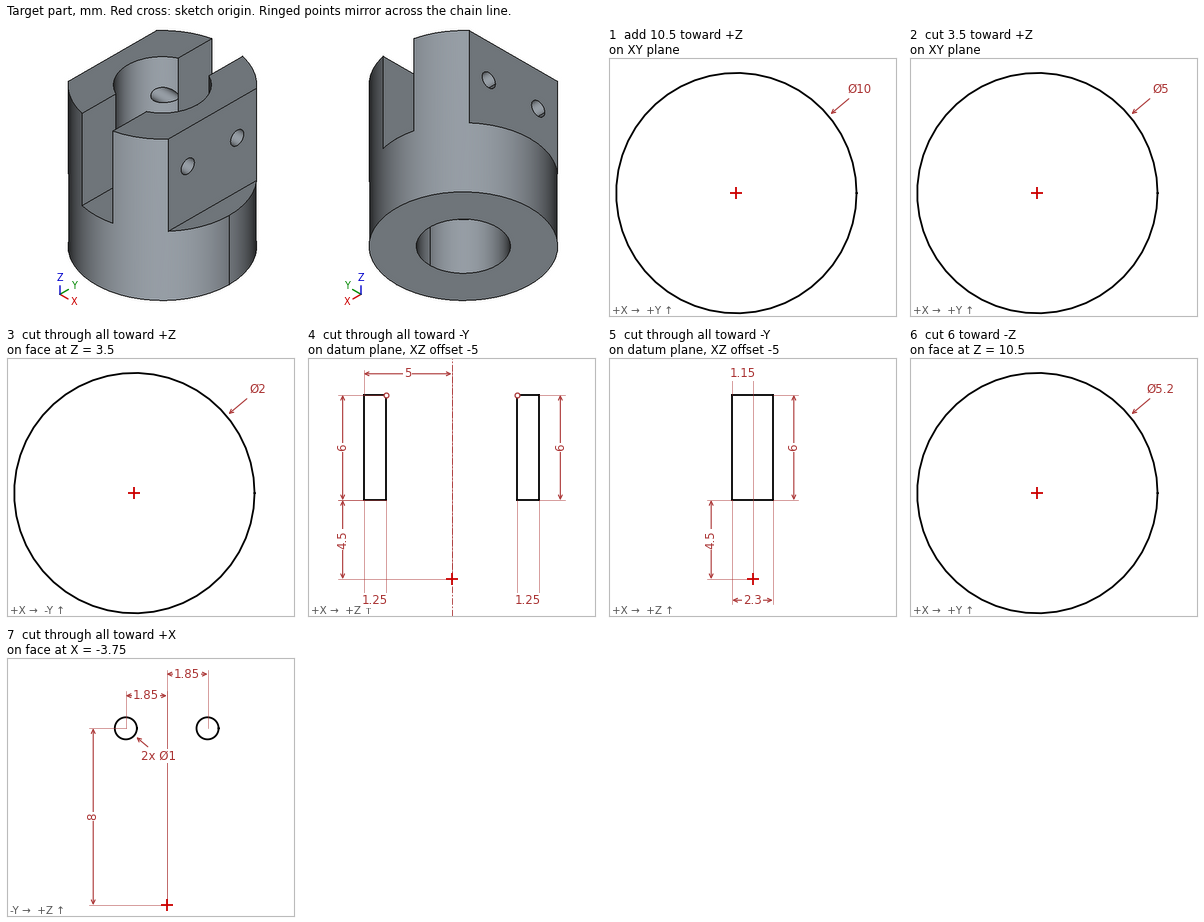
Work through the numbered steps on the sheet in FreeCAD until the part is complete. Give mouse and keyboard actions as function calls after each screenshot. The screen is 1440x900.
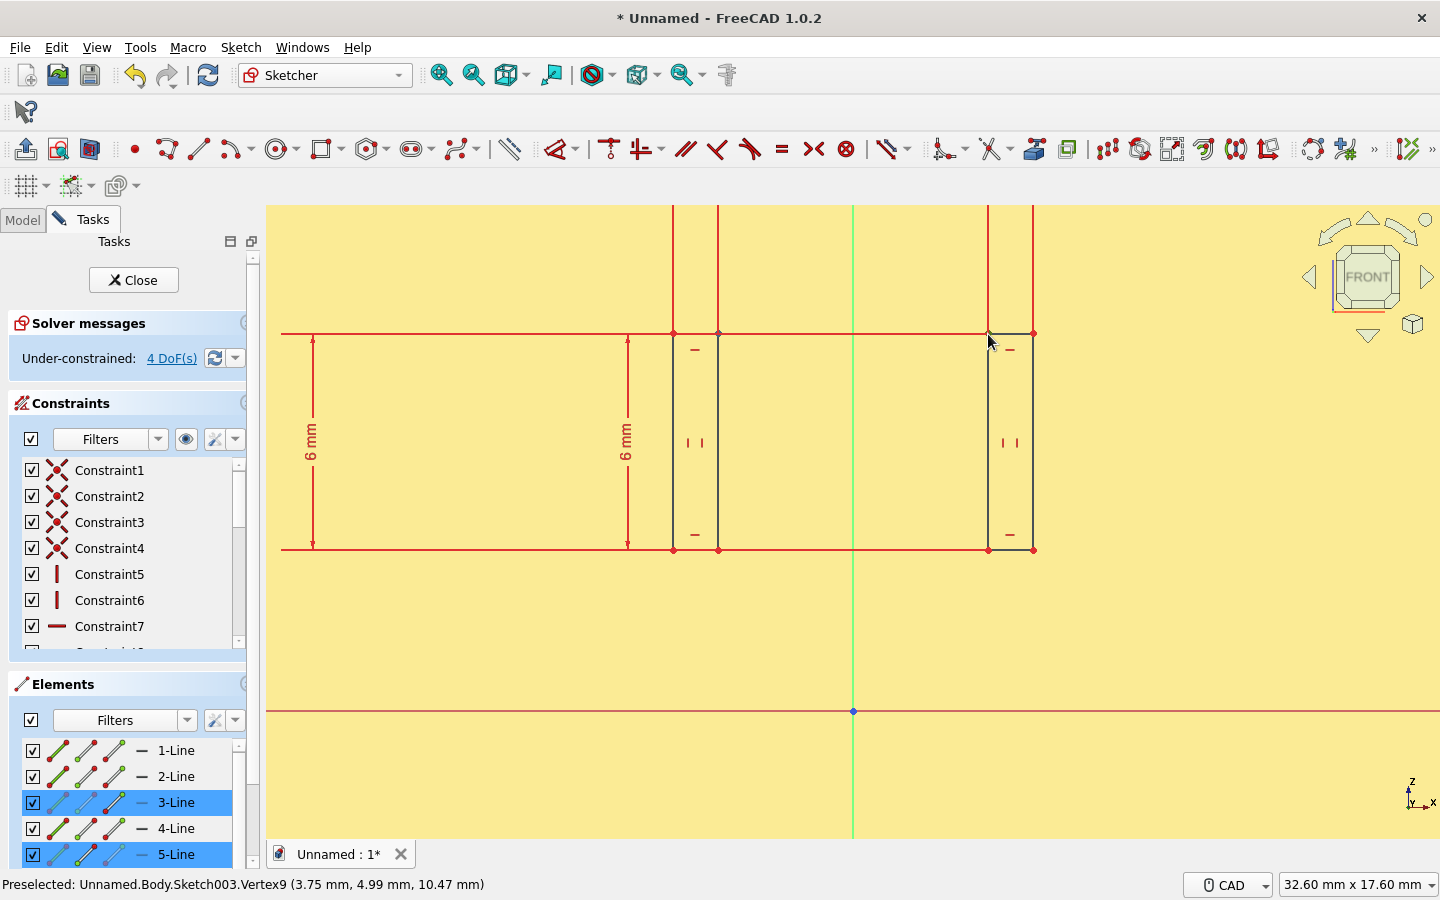
click(853, 770)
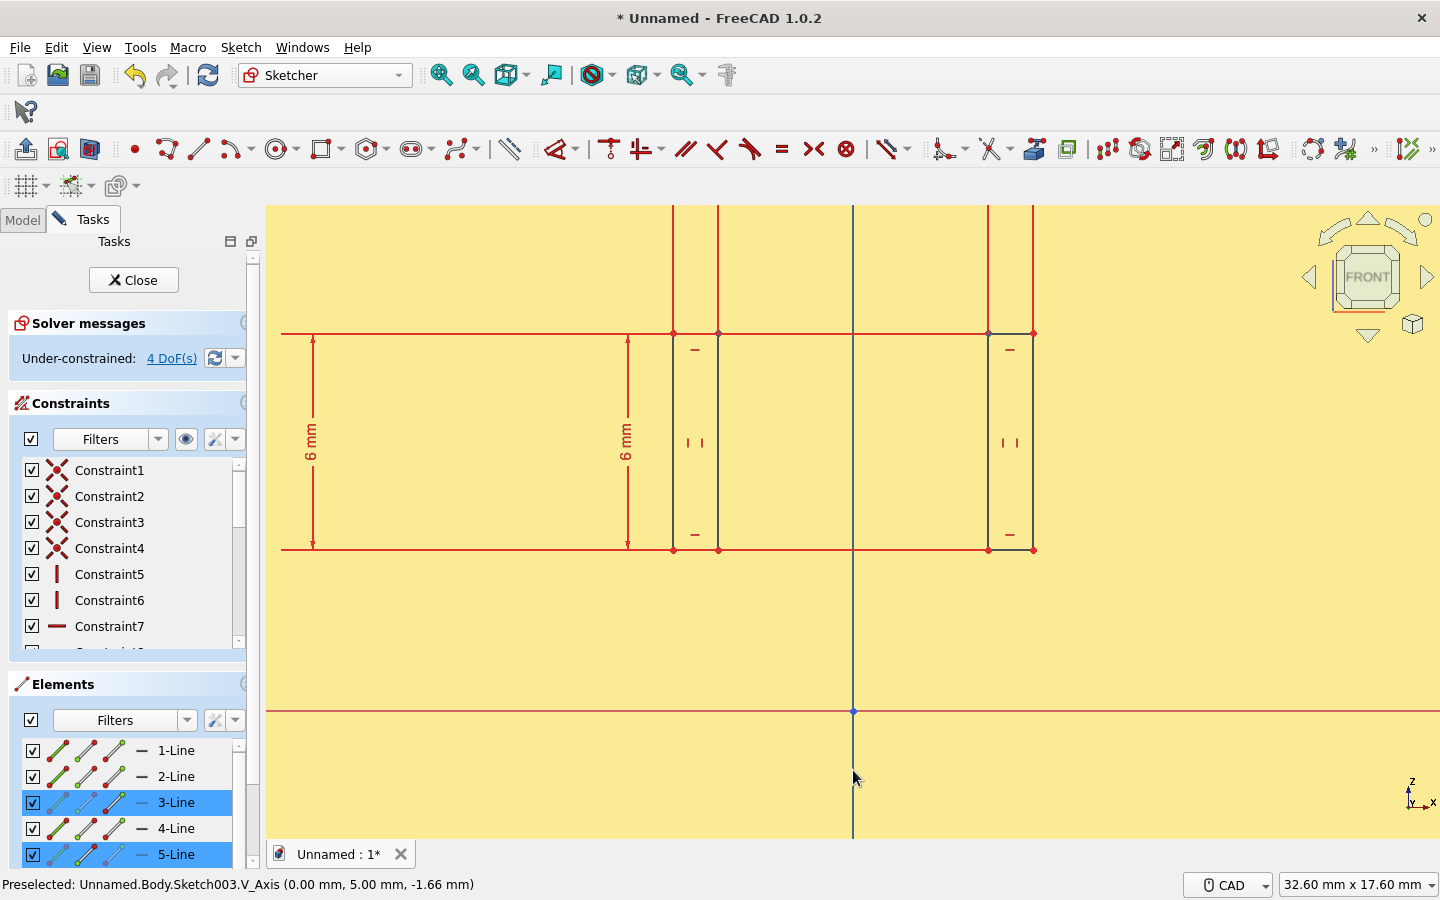
key(s)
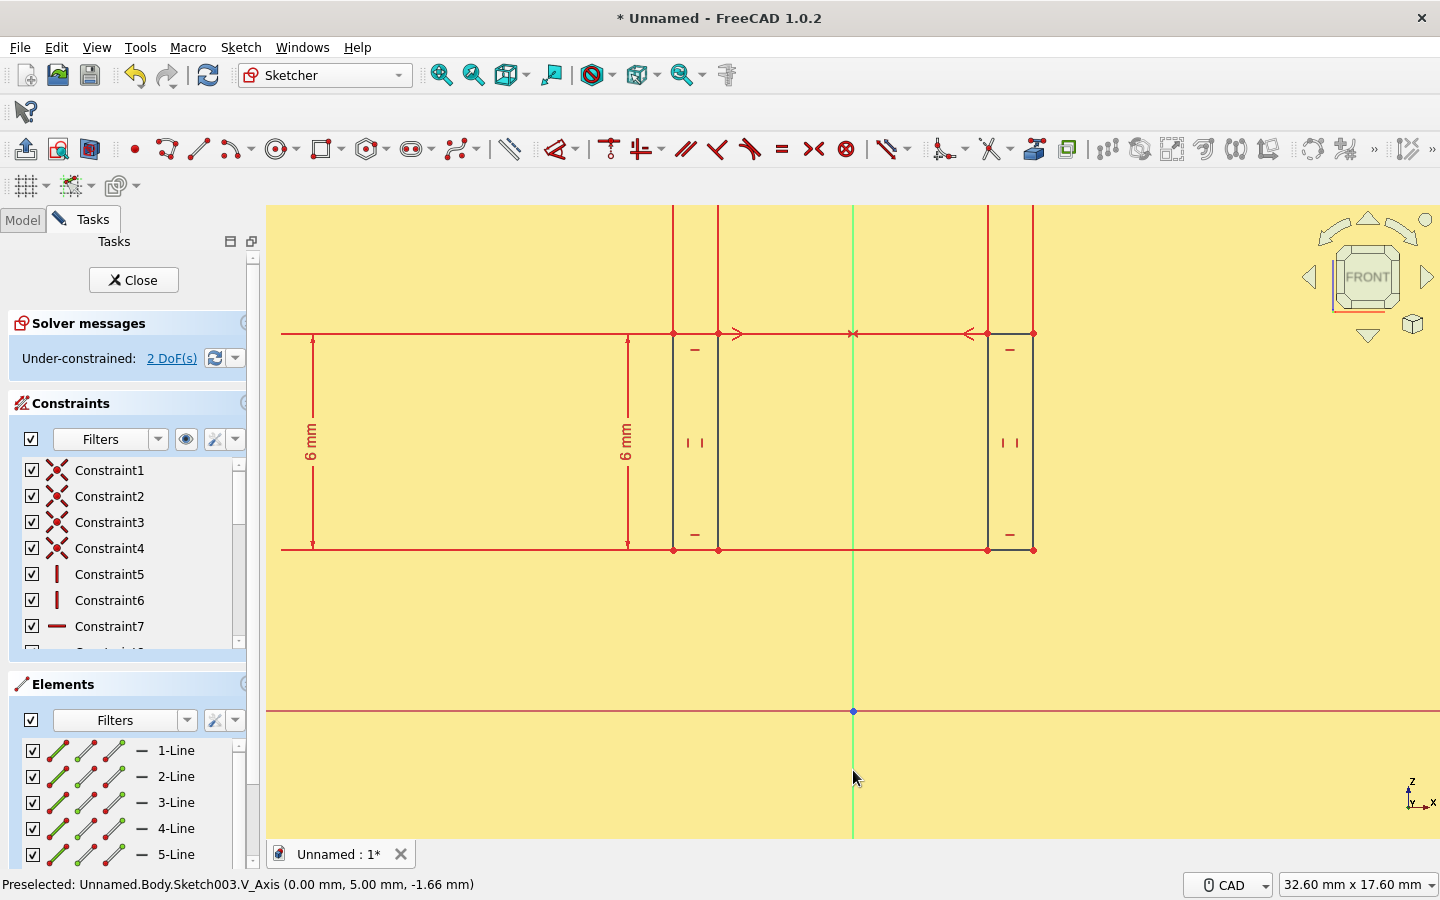
click(673, 334)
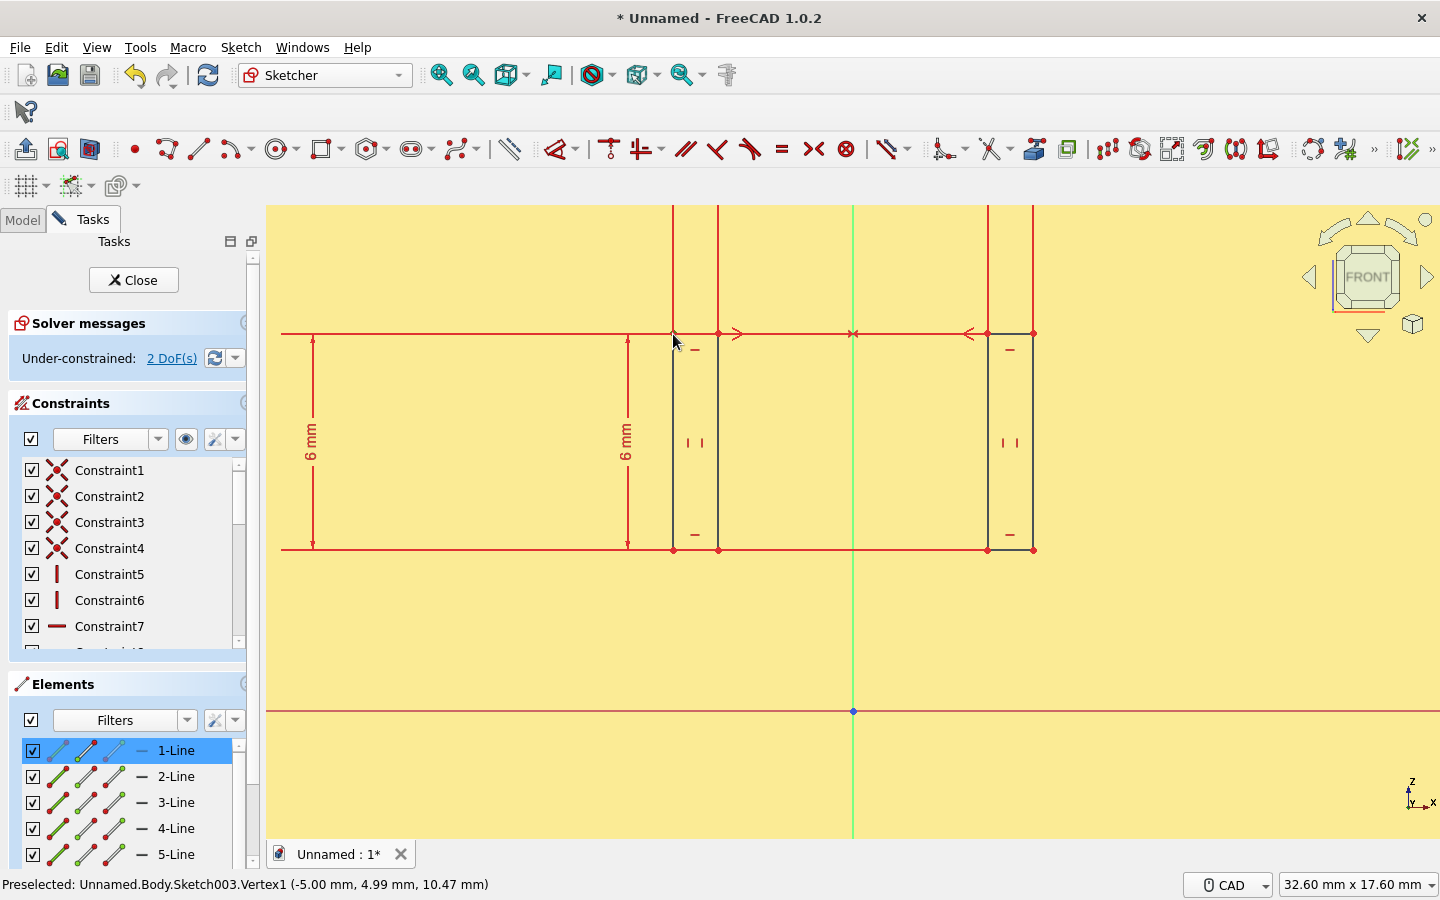
click(578, 150)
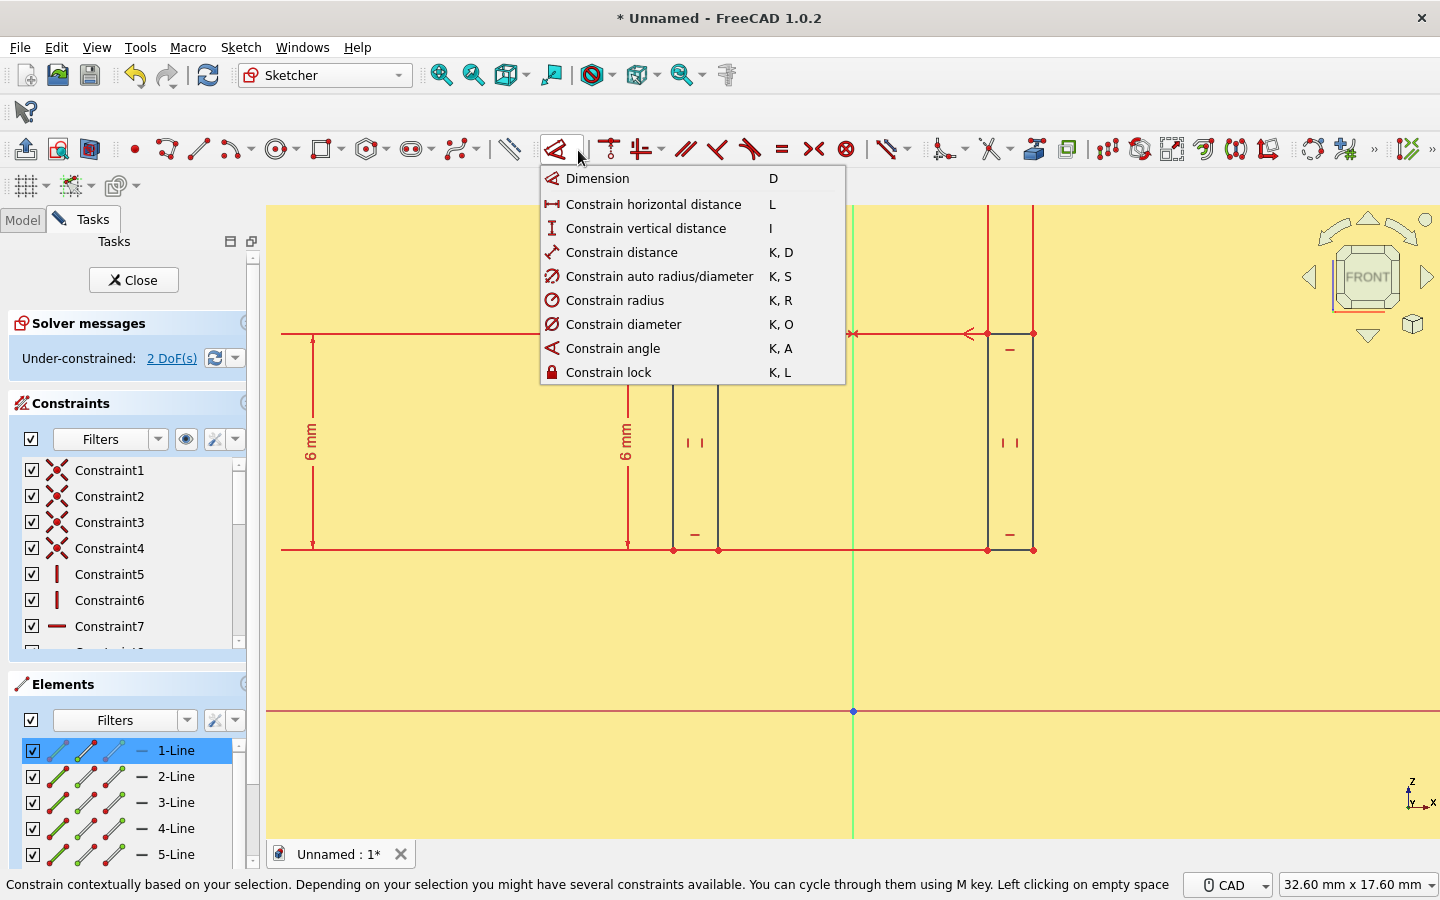
click(693, 204)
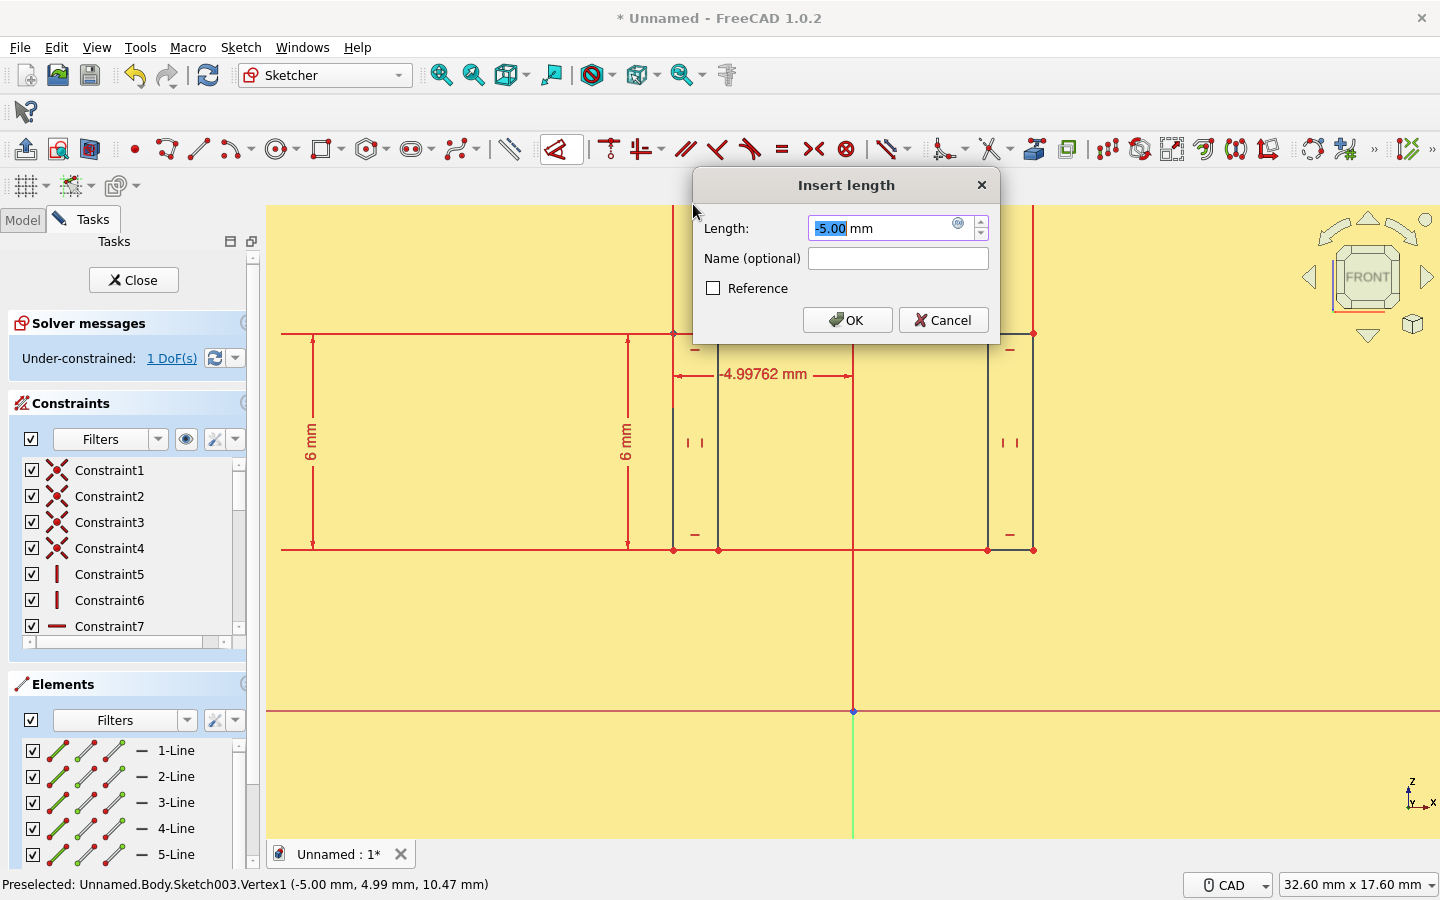
text(-5)
key(Return)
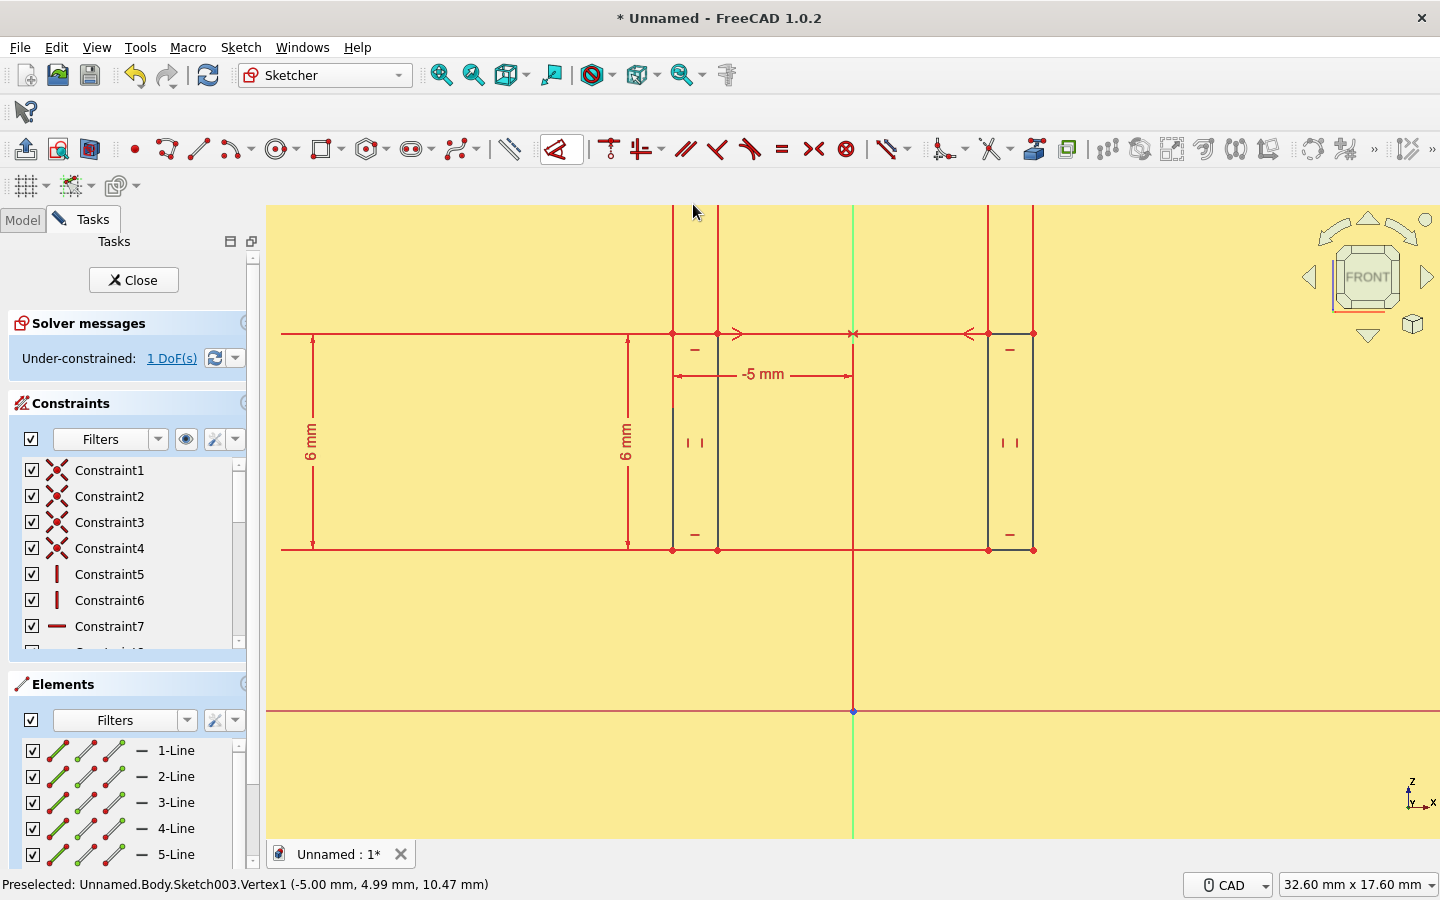
click(673, 550)